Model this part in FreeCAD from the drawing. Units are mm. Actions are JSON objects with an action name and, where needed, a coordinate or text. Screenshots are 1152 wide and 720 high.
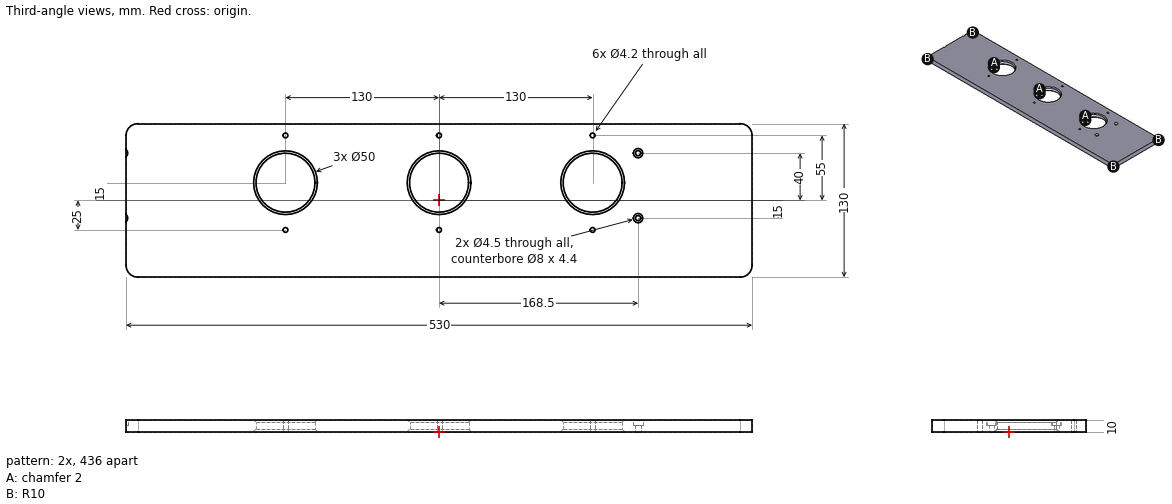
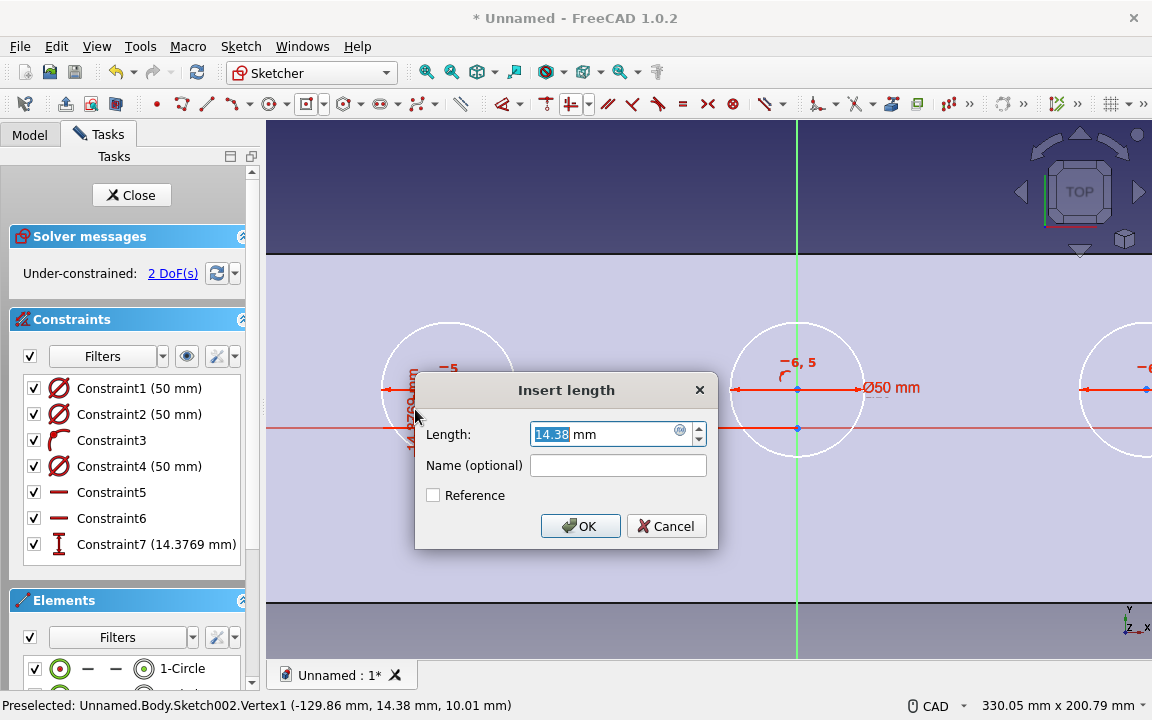
{"action": "type", "text": "15"}
{"action": "key", "text": "Return"}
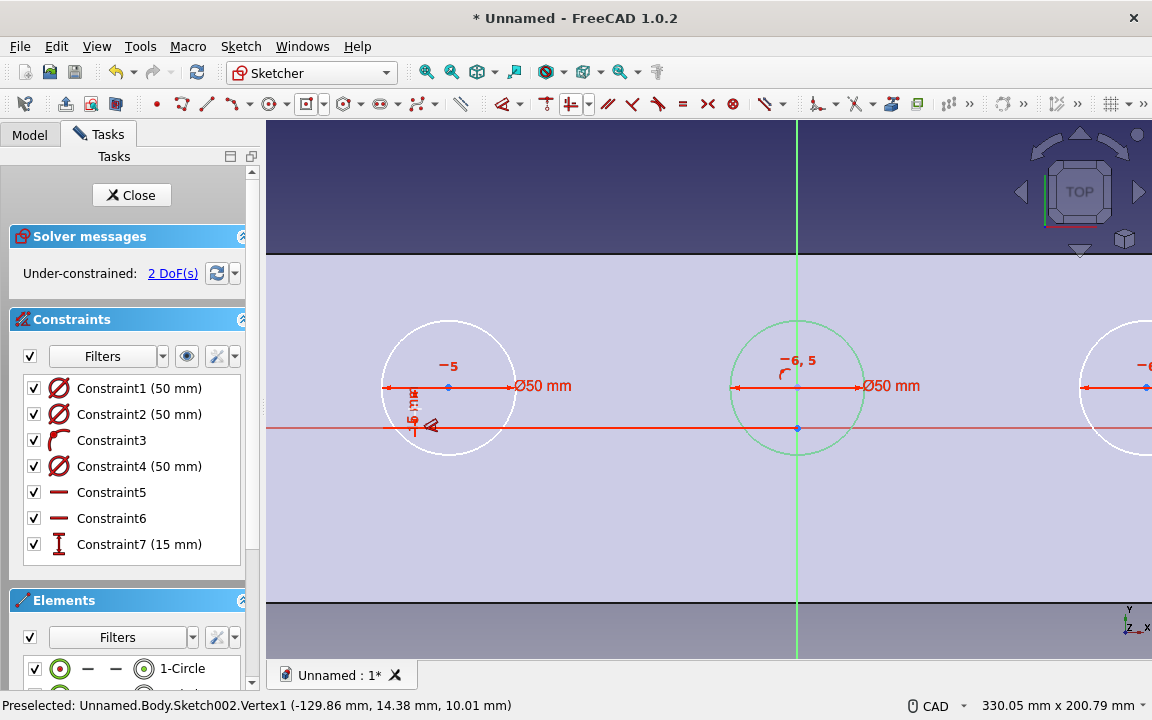
{"action": "left_click", "coordinate": [449, 388]}
{"action": "left_click", "coordinate": [623, 462]}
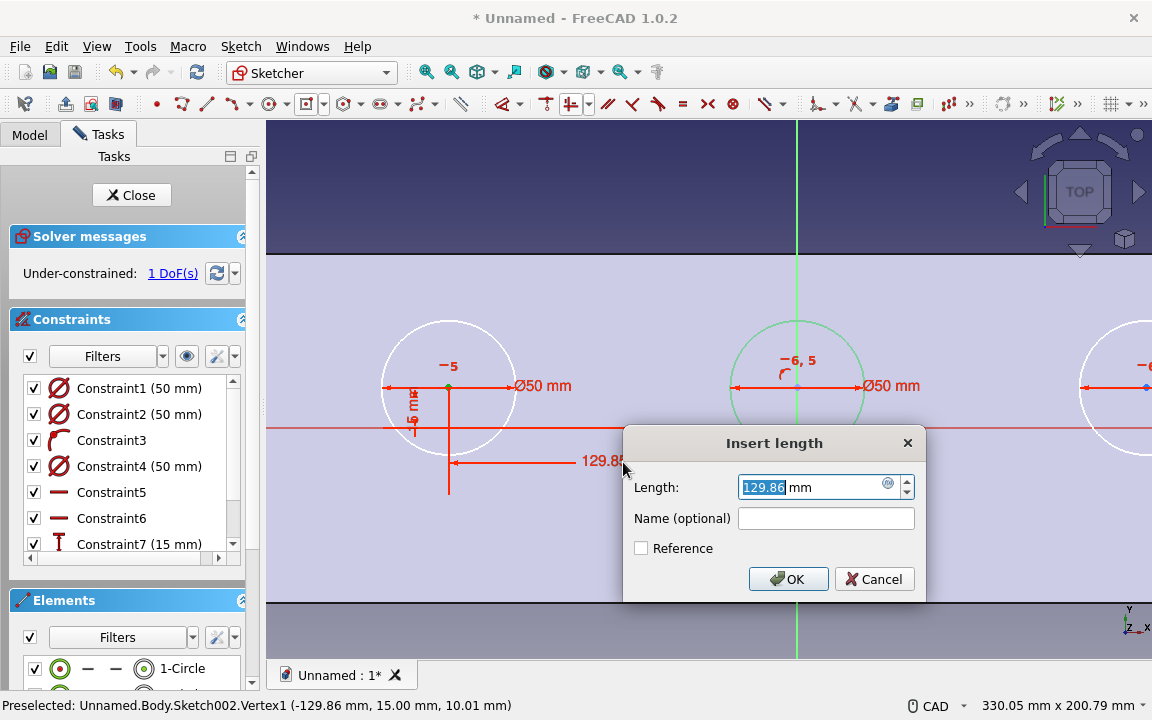
{"action": "type", "text": "130"}
{"action": "key", "text": "Return"}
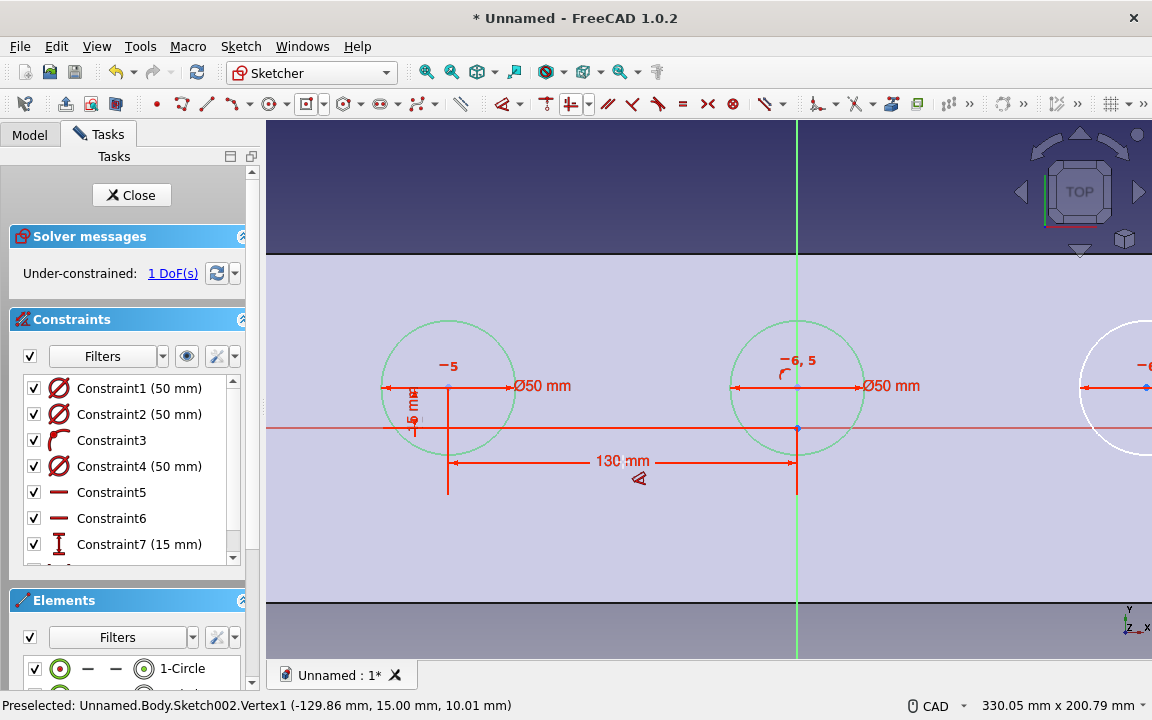
{"action": "scroll", "coordinate": [450, 391], "scroll_direction": "down", "scroll_amount": 3}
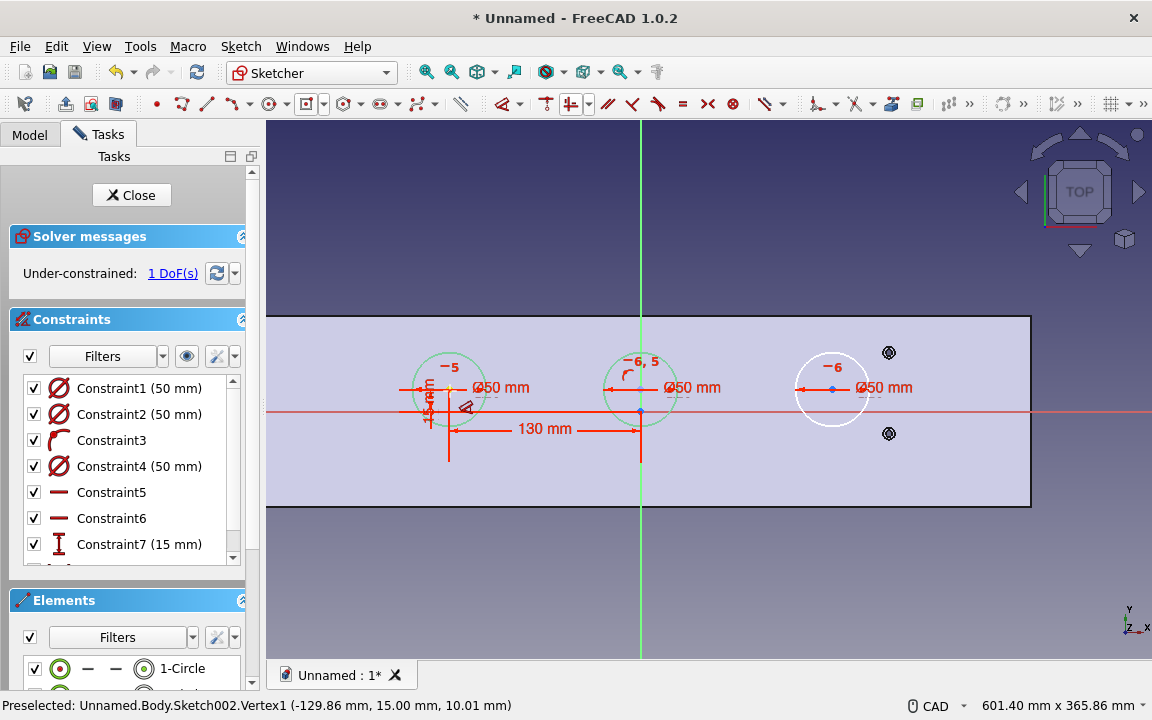
{"action": "left_click", "coordinate": [832, 390]}
{"action": "left_click", "coordinate": [737, 446]}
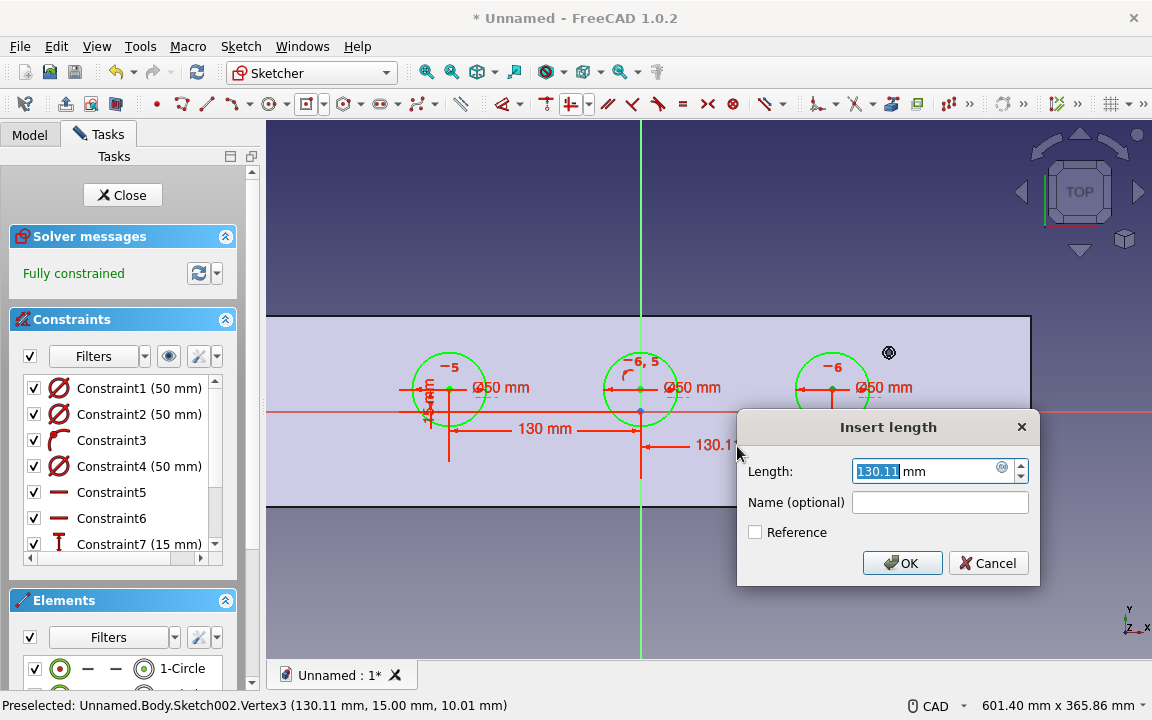
{"action": "type", "text": "130"}
{"action": "key", "text": "Return"}
{"action": "key", "text": "Escape"}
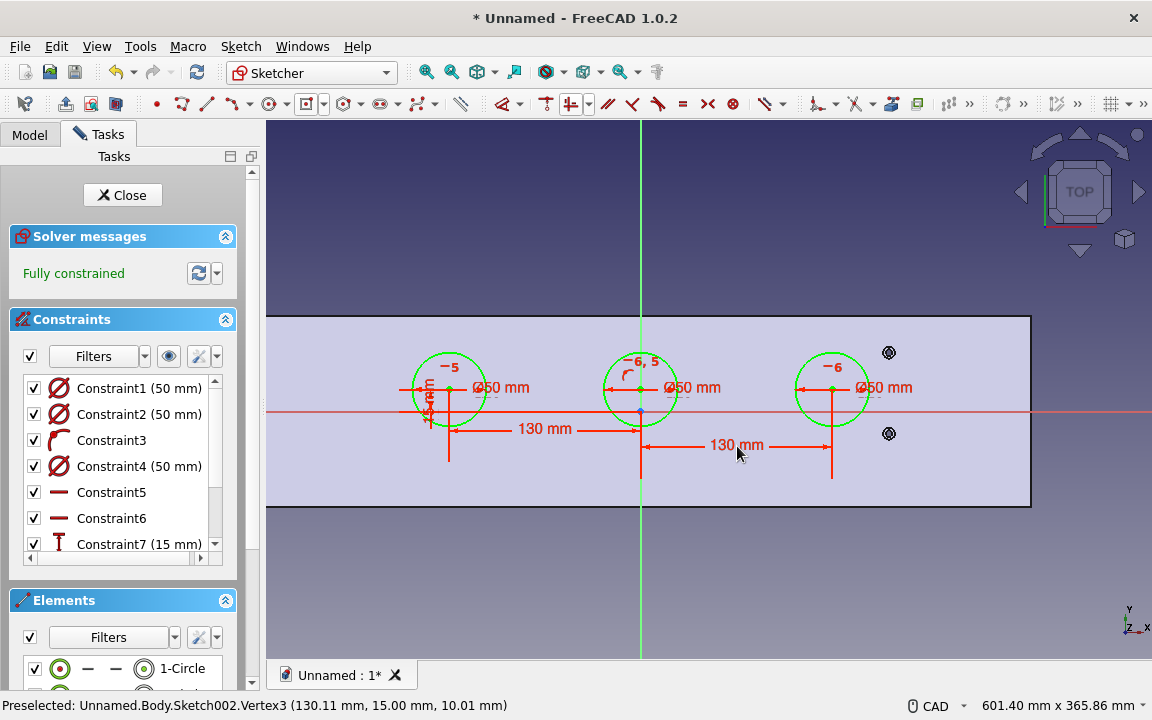
{"action": "left_click", "coordinate": [123, 195]}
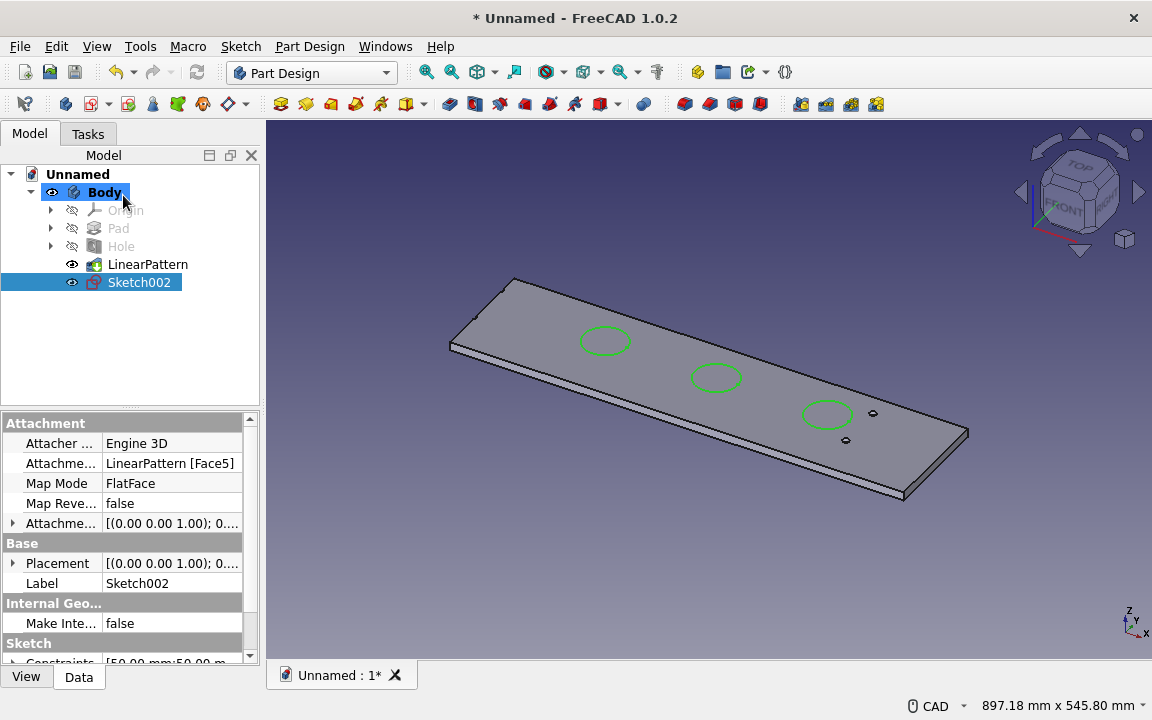
{"action": "left_click", "coordinate": [450, 104]}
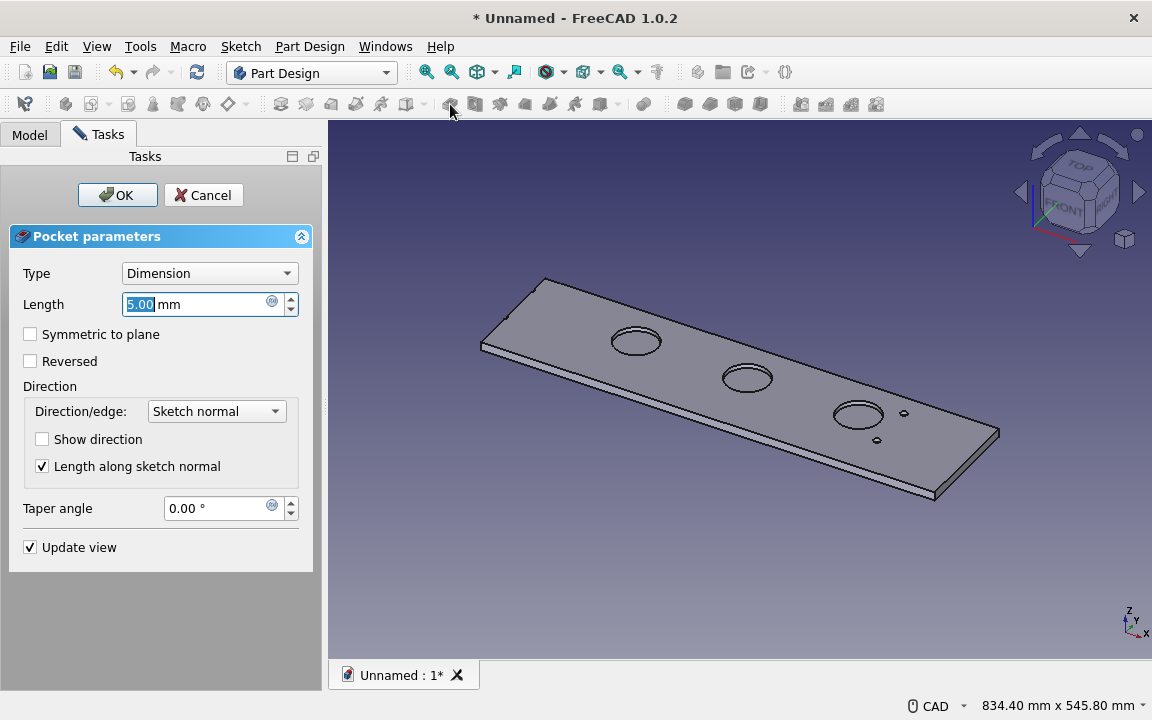
{"action": "left_click", "coordinate": [210, 274]}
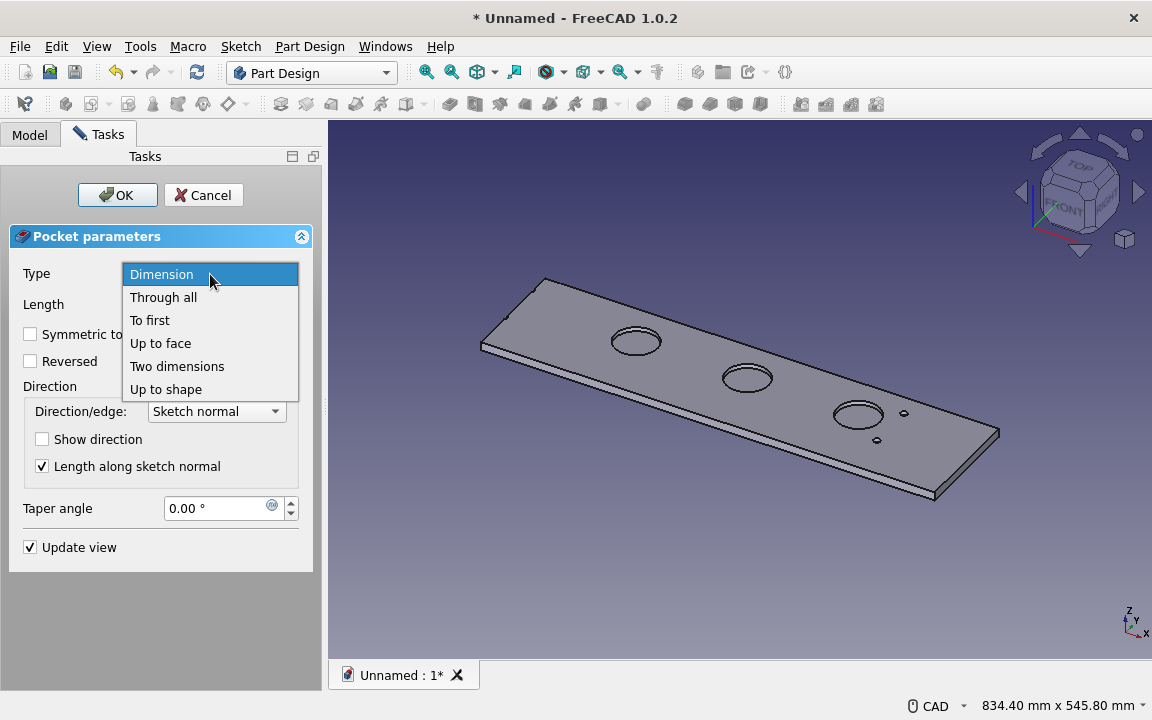
{"action": "left_click", "coordinate": [208, 298]}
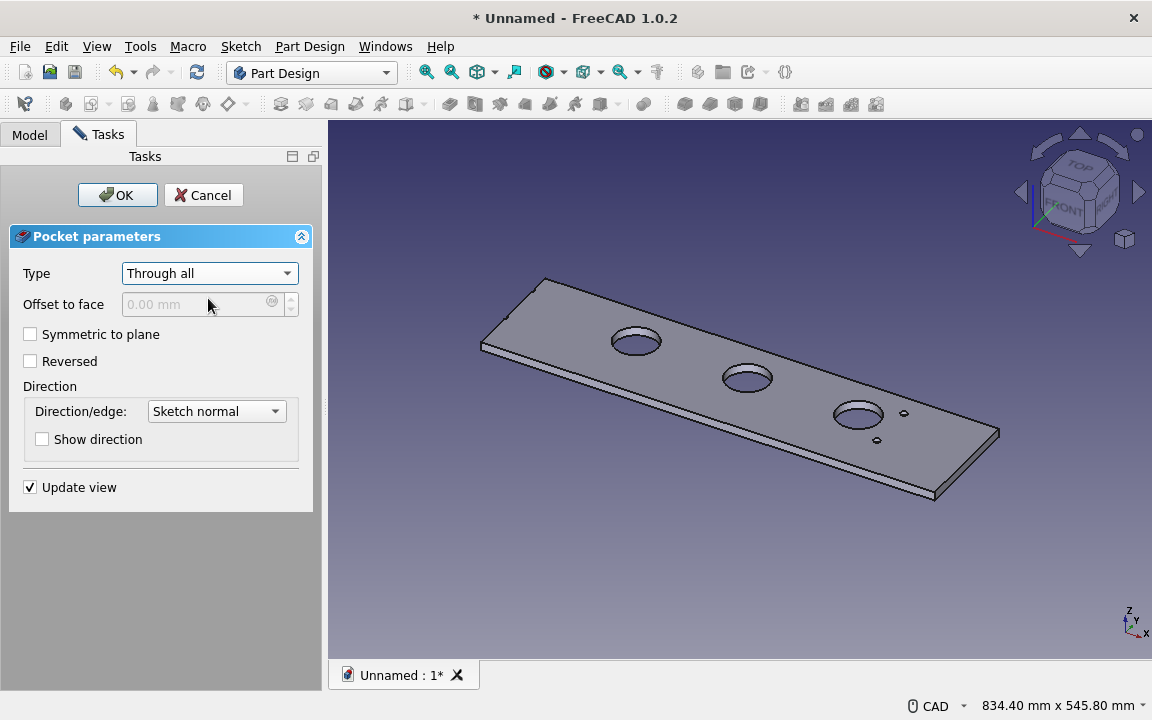
{"action": "left_click", "coordinate": [118, 195]}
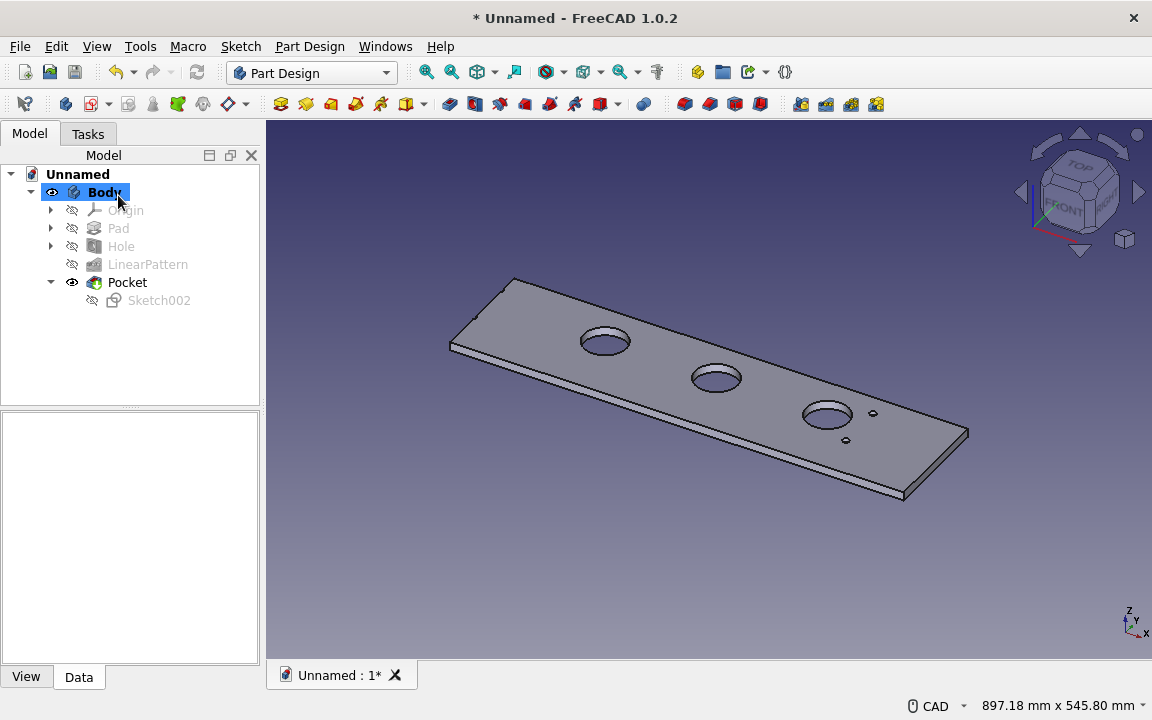
{"action": "left_click", "coordinate": [584, 333]}